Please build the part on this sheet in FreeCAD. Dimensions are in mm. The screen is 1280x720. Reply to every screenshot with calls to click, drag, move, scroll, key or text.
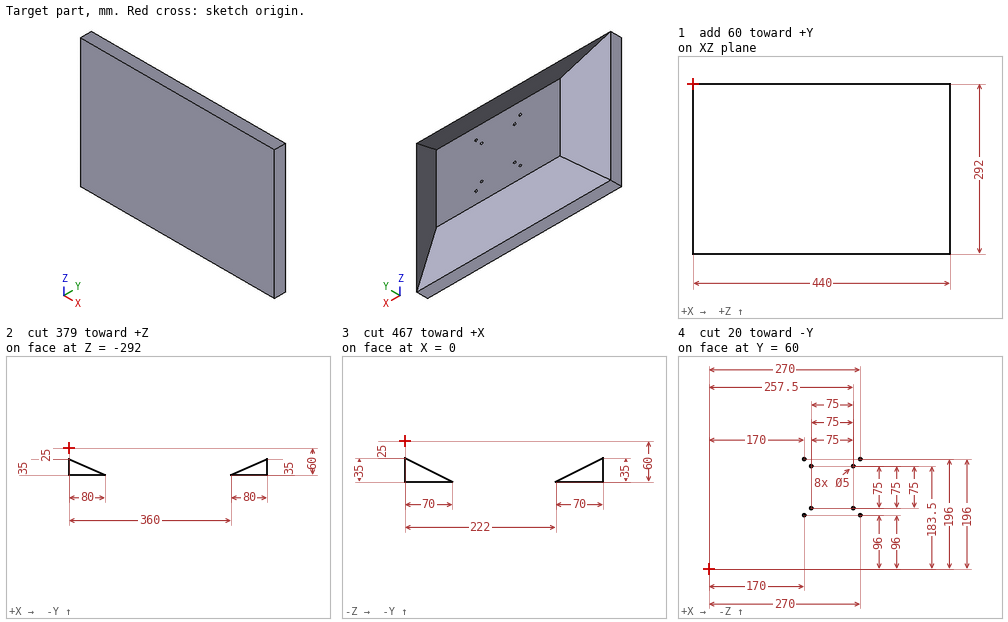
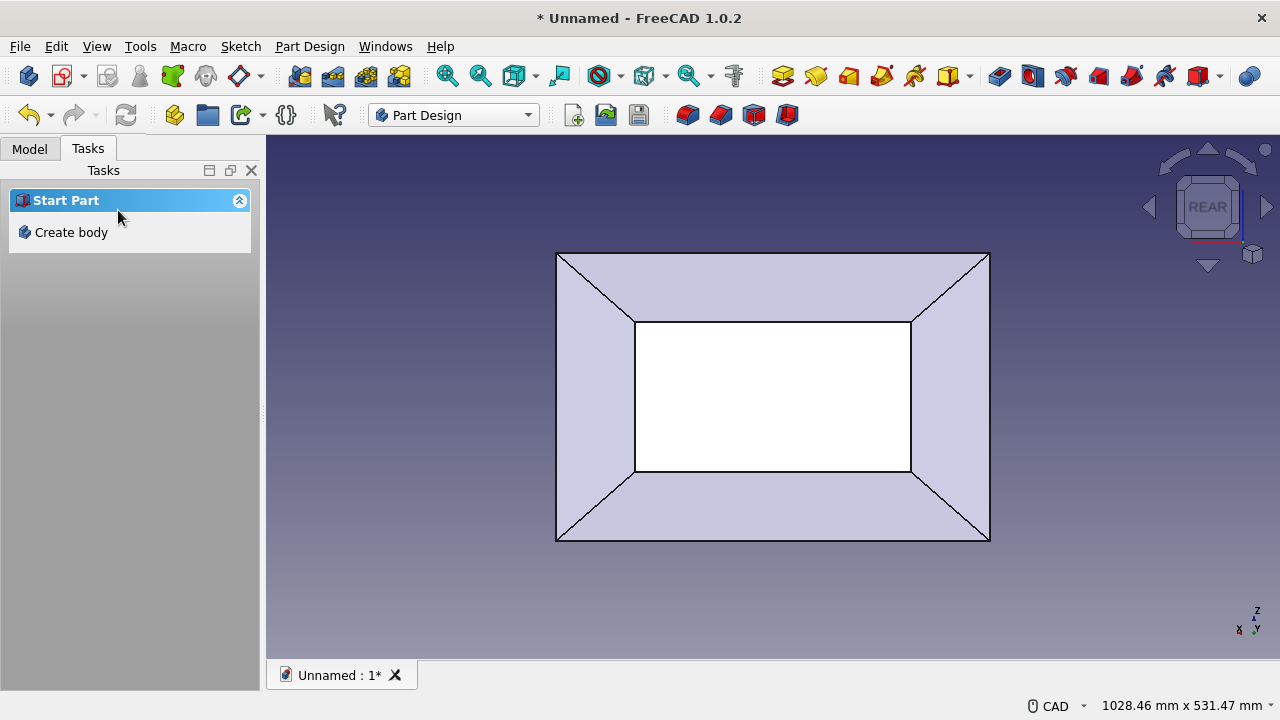
click(734, 396)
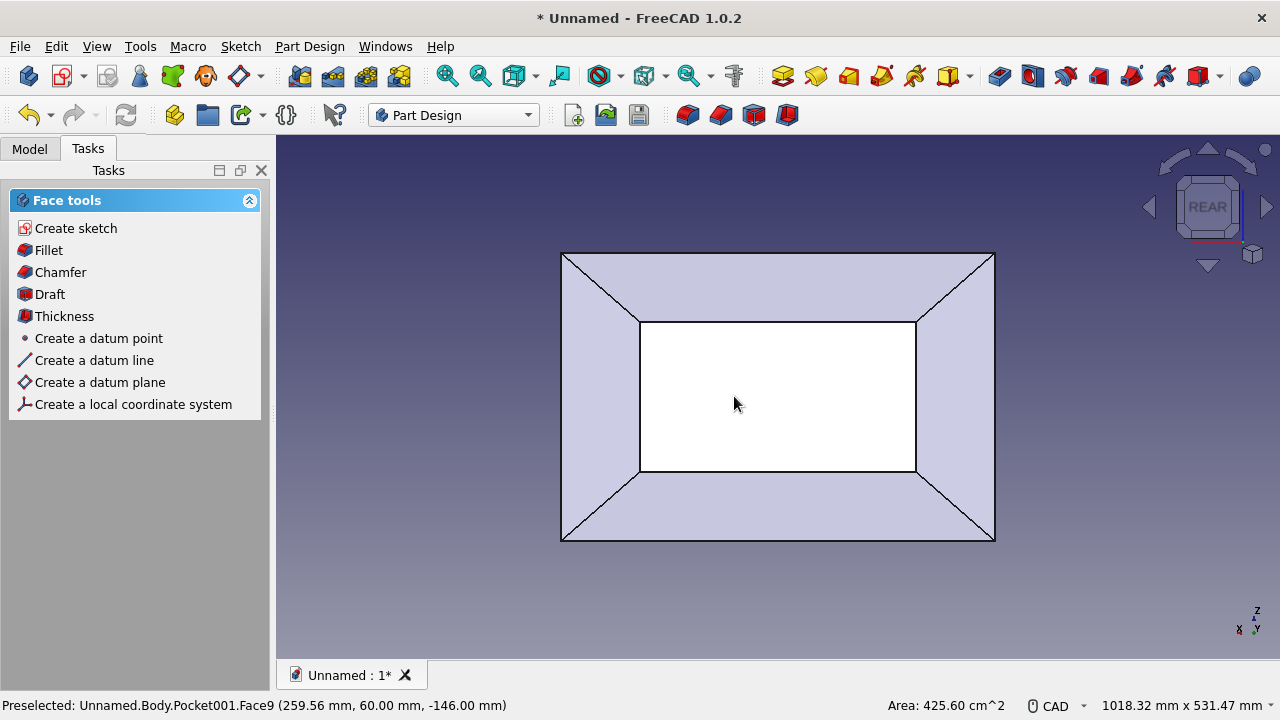
click(62, 76)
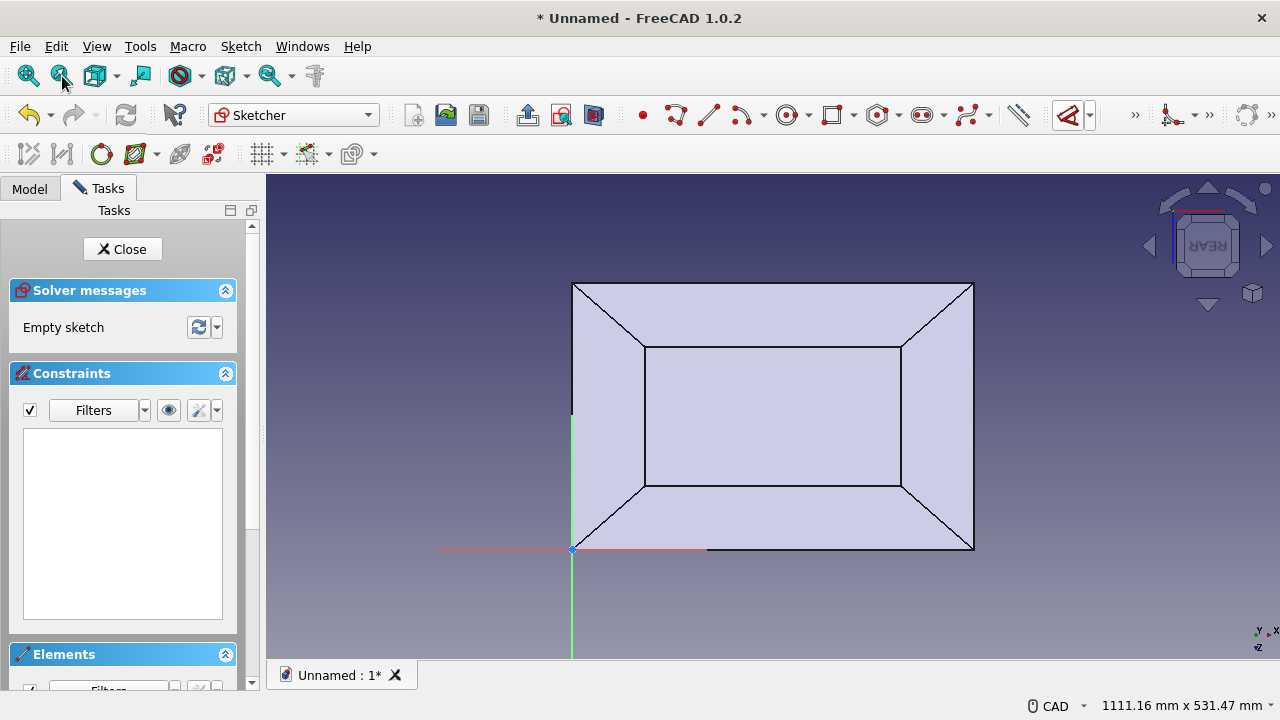
scroll(803, 416, up, 6)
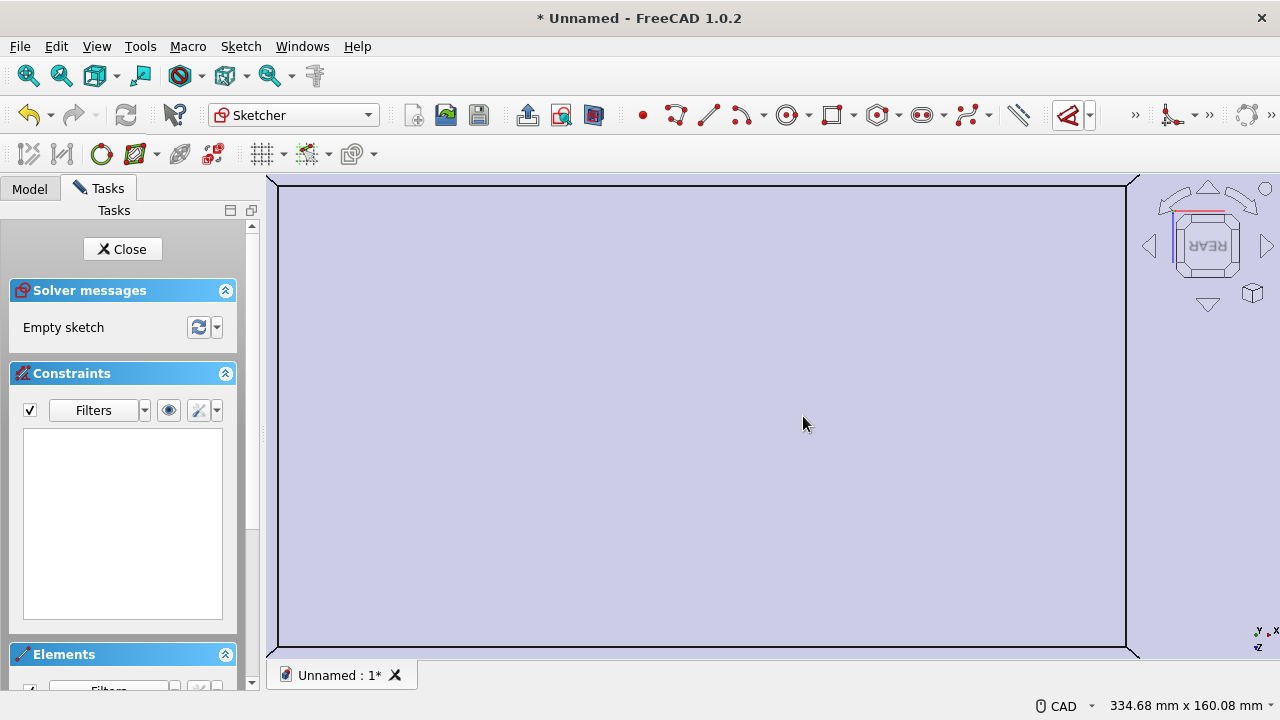
click(786, 116)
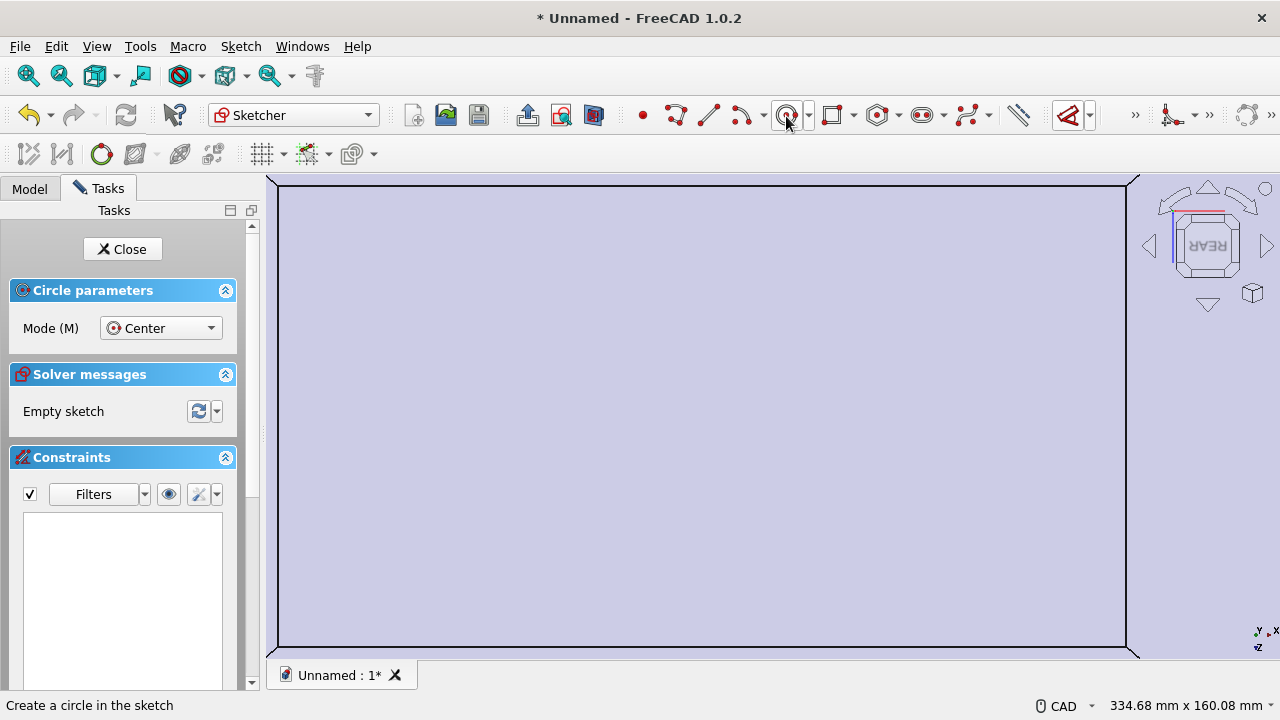
scroll(854, 265, up, 6)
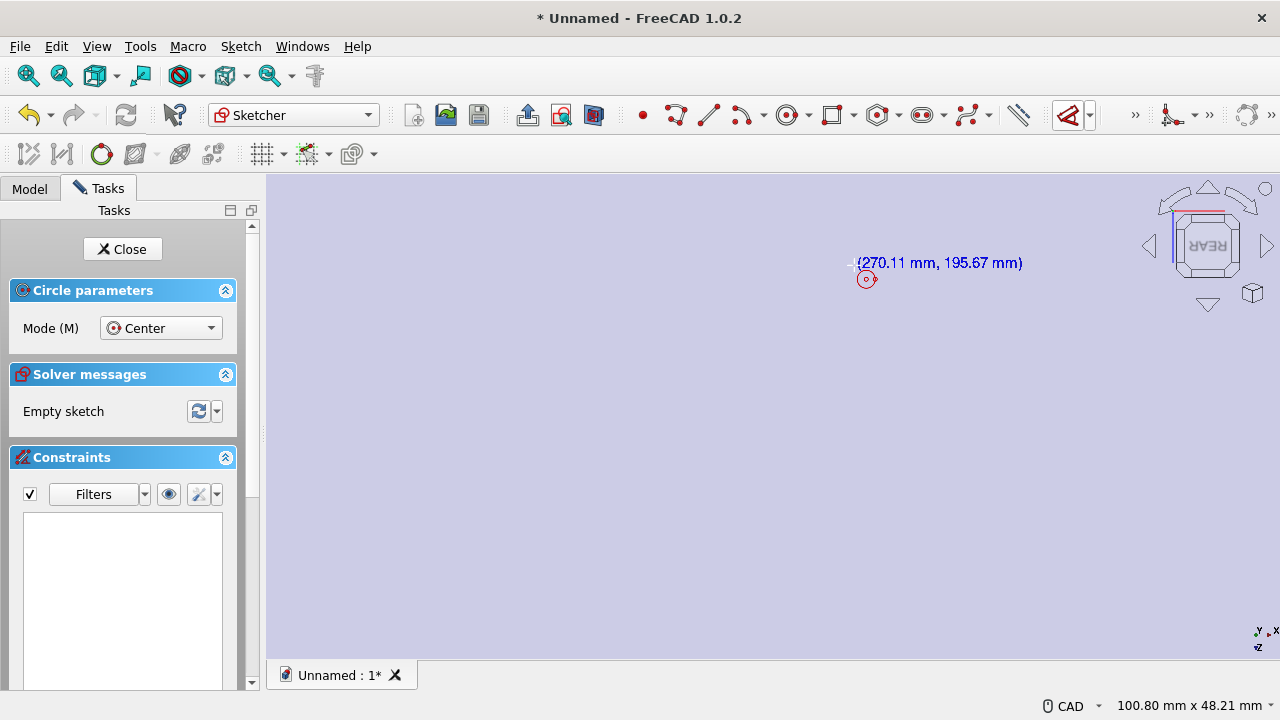
click(852, 265)
move(869, 247)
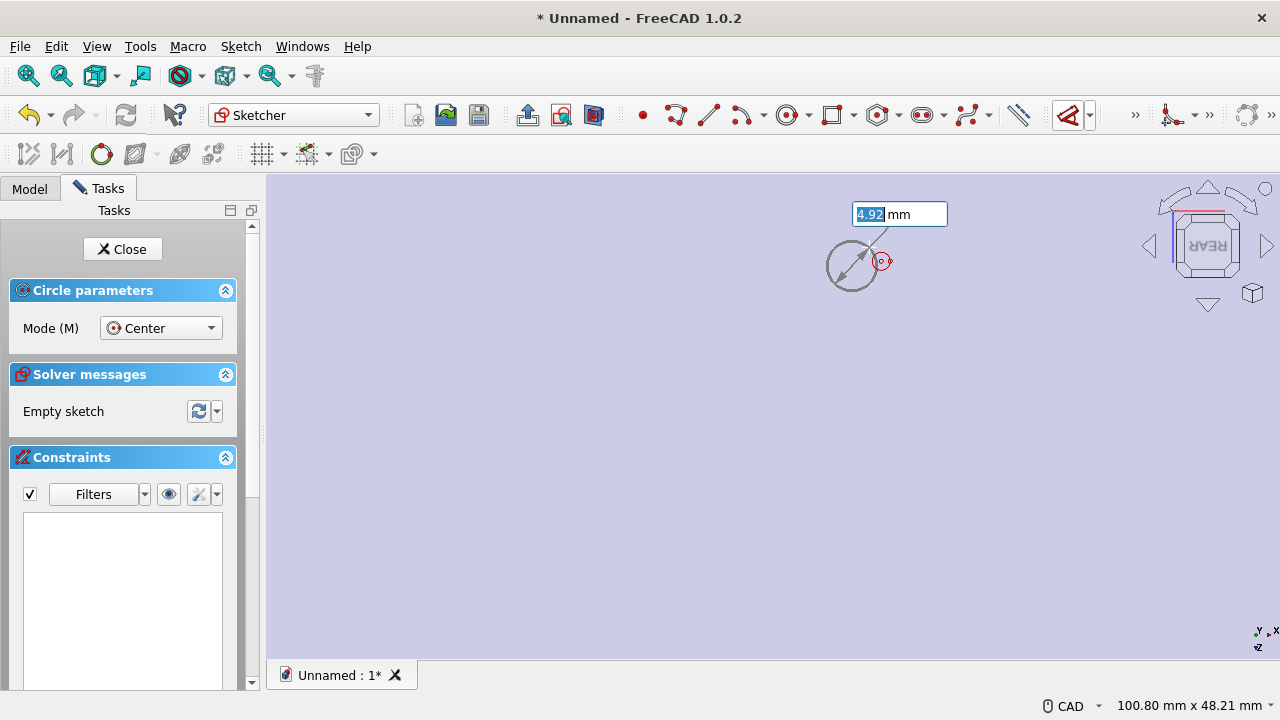
text(5)
key(Return)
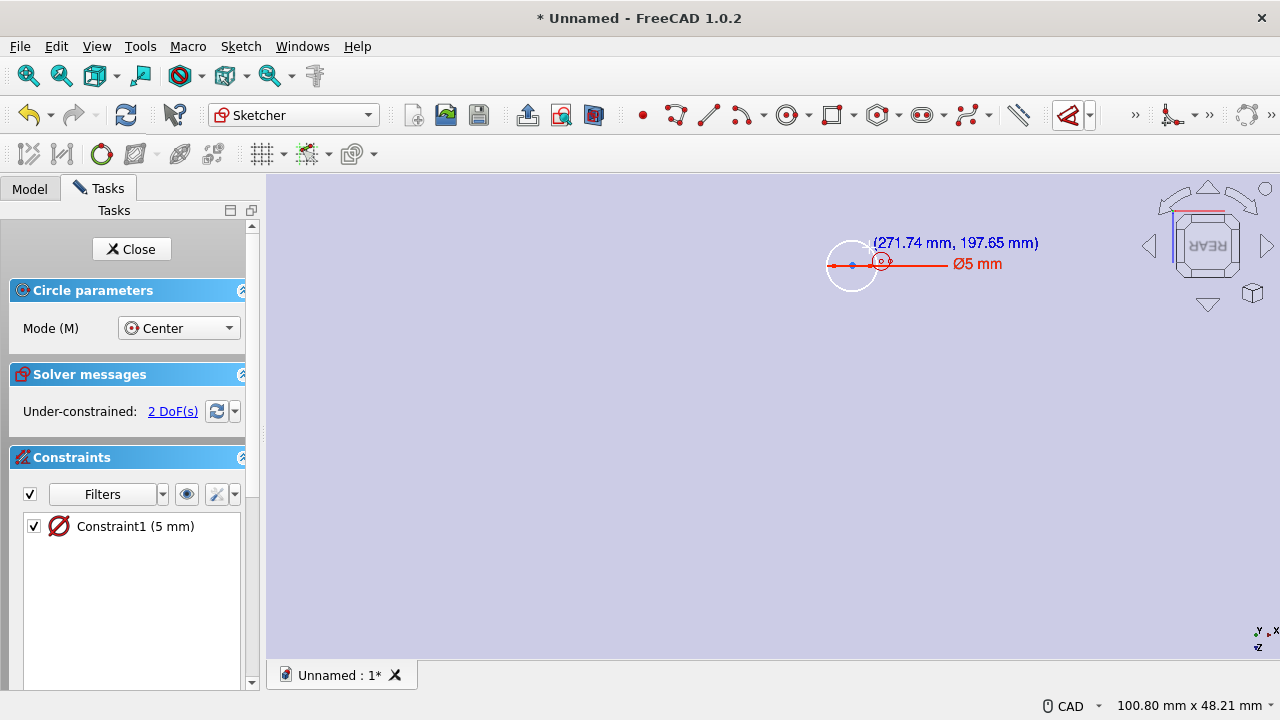
click(726, 390)
move(744, 373)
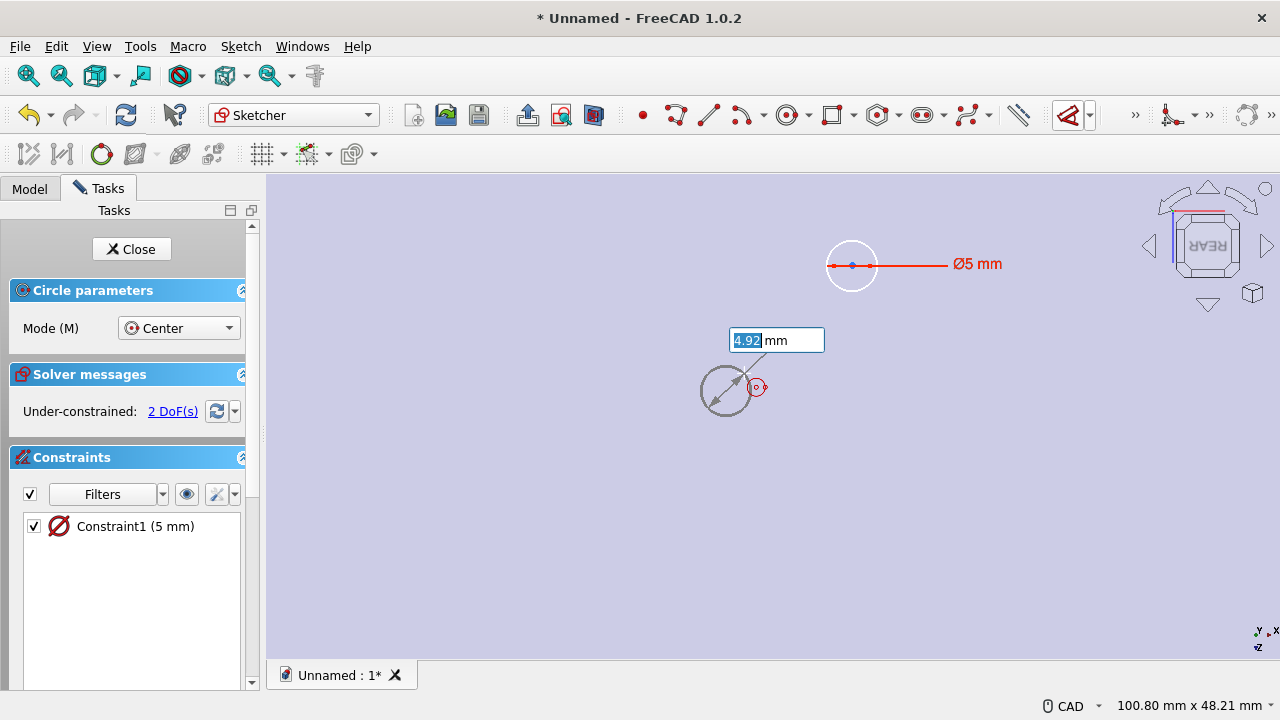
text(5)
key(Return)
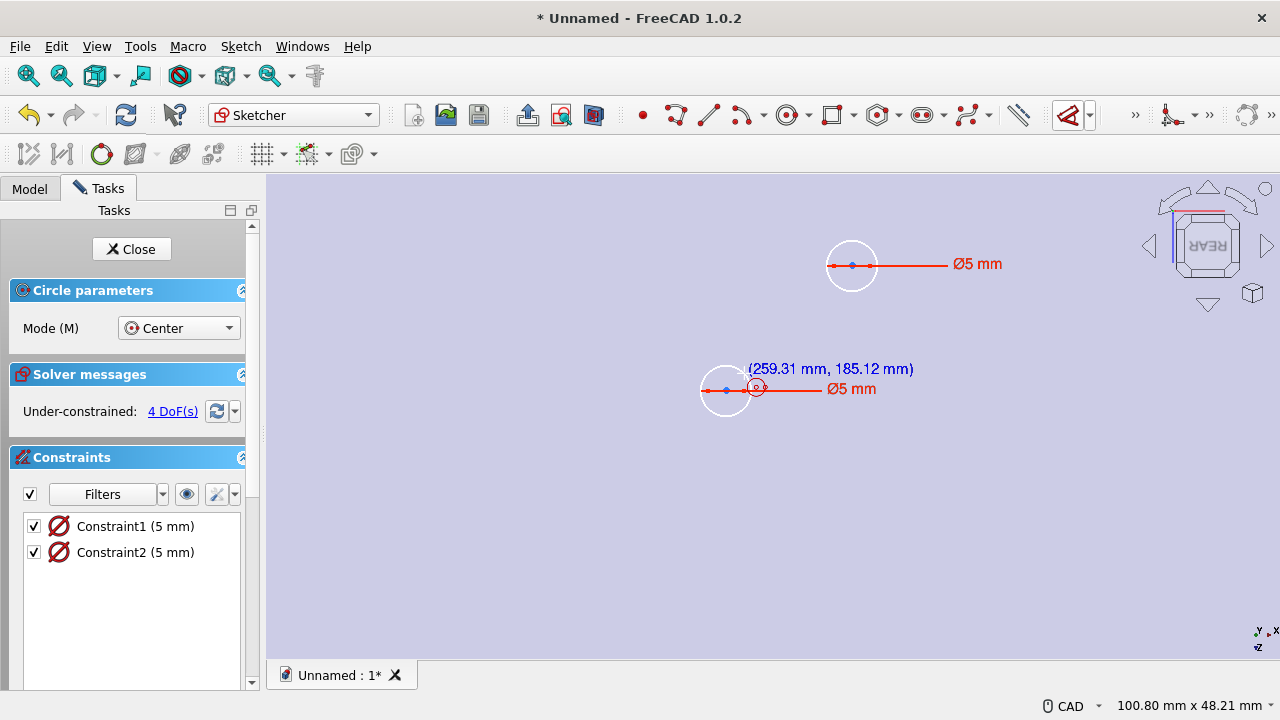
scroll(858, 265, down, 6)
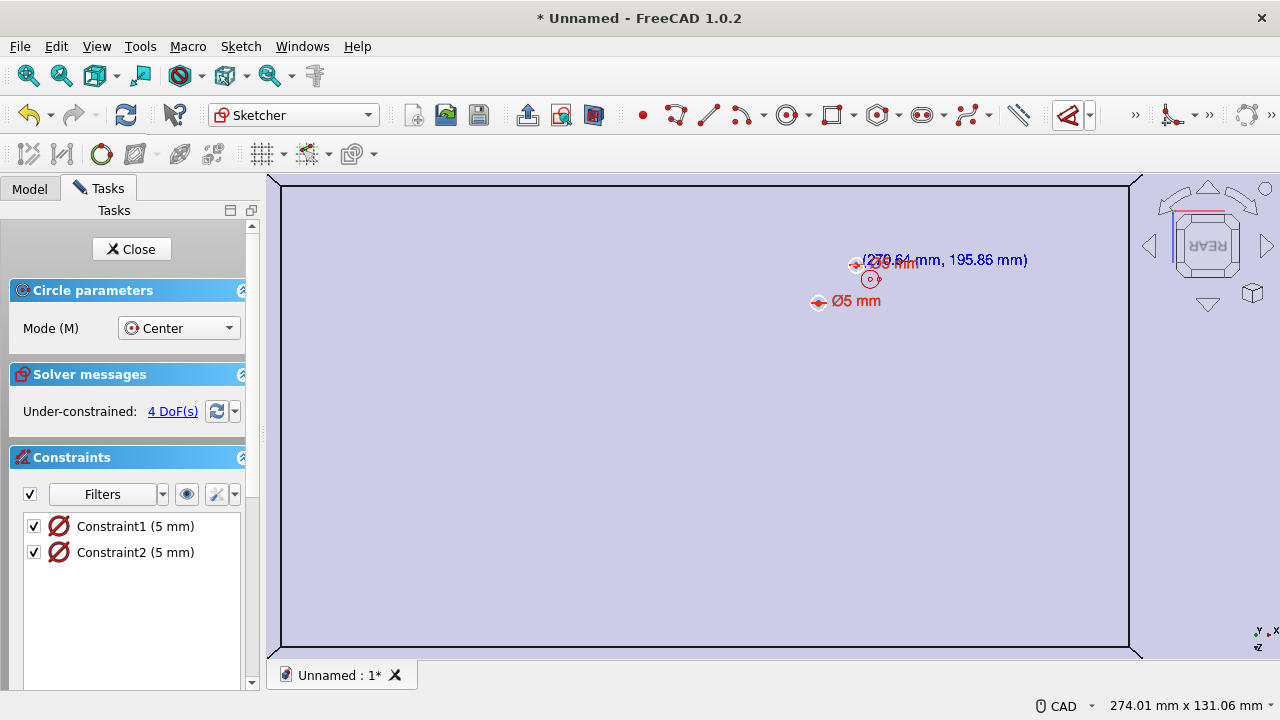
scroll(856, 568, up, 6)